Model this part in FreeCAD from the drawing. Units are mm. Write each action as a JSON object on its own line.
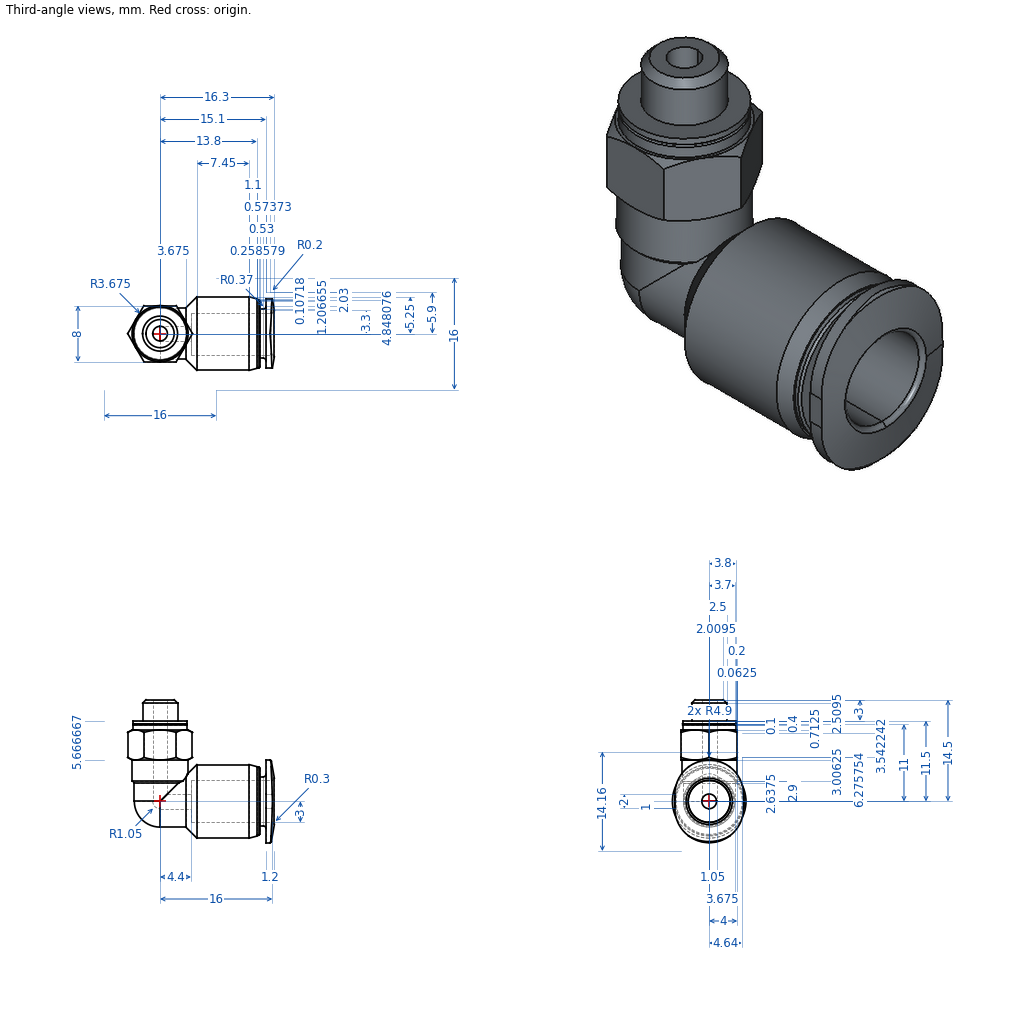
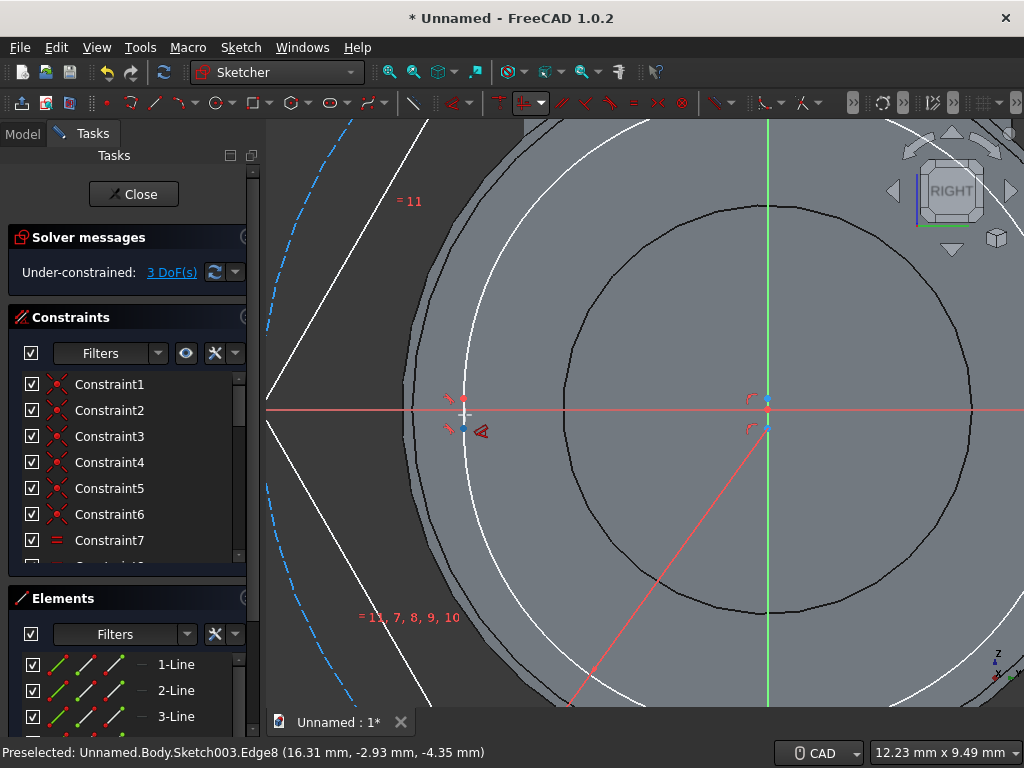
{"action": "left_click", "coordinate": [464, 414]}
{"action": "left_click", "coordinate": [430, 424]}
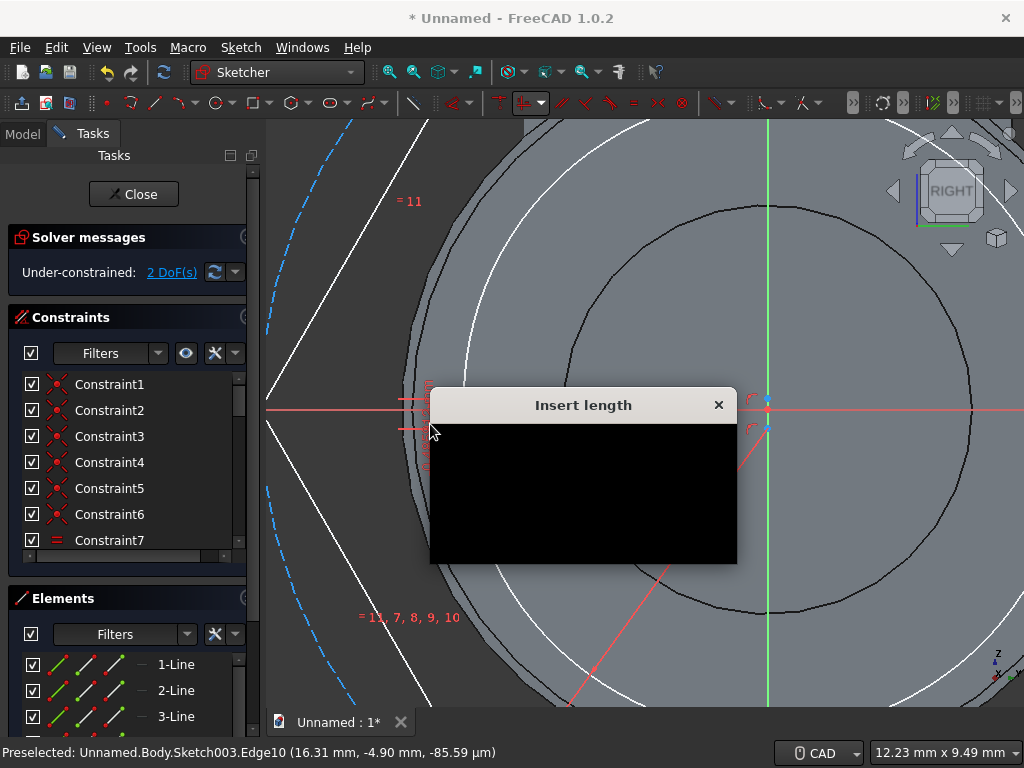
{"action": "type", "text": "2"}
{"action": "key", "text": "Return"}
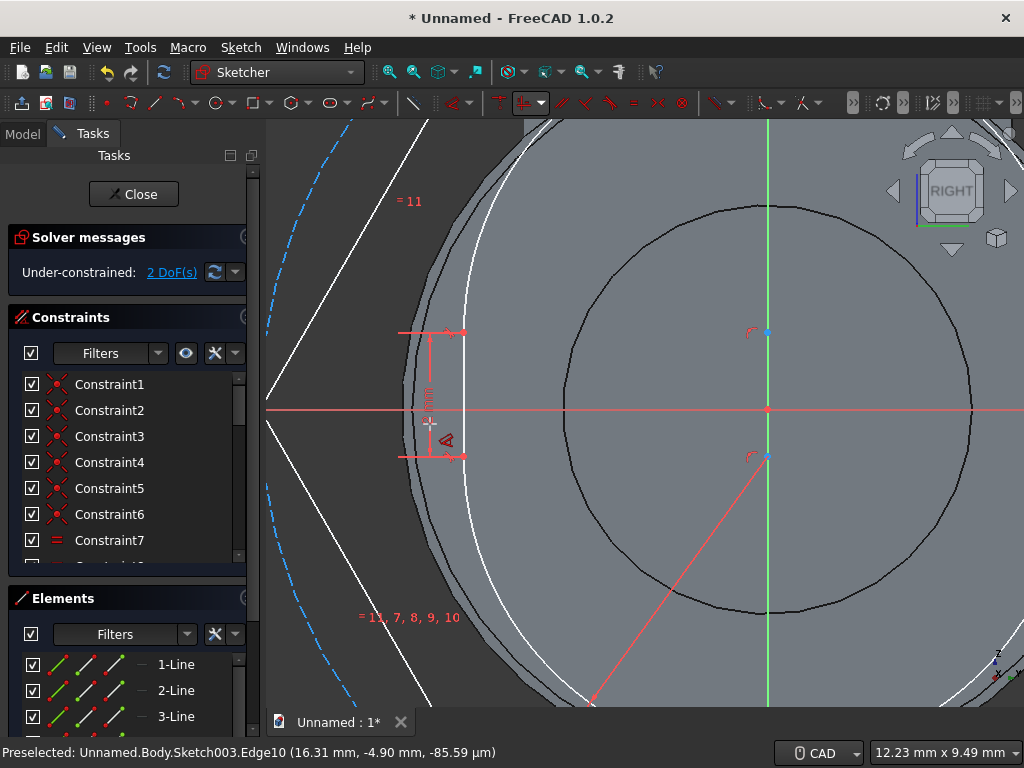
{"action": "left_click", "coordinate": [464, 457]}
{"action": "left_click", "coordinate": [430, 450]}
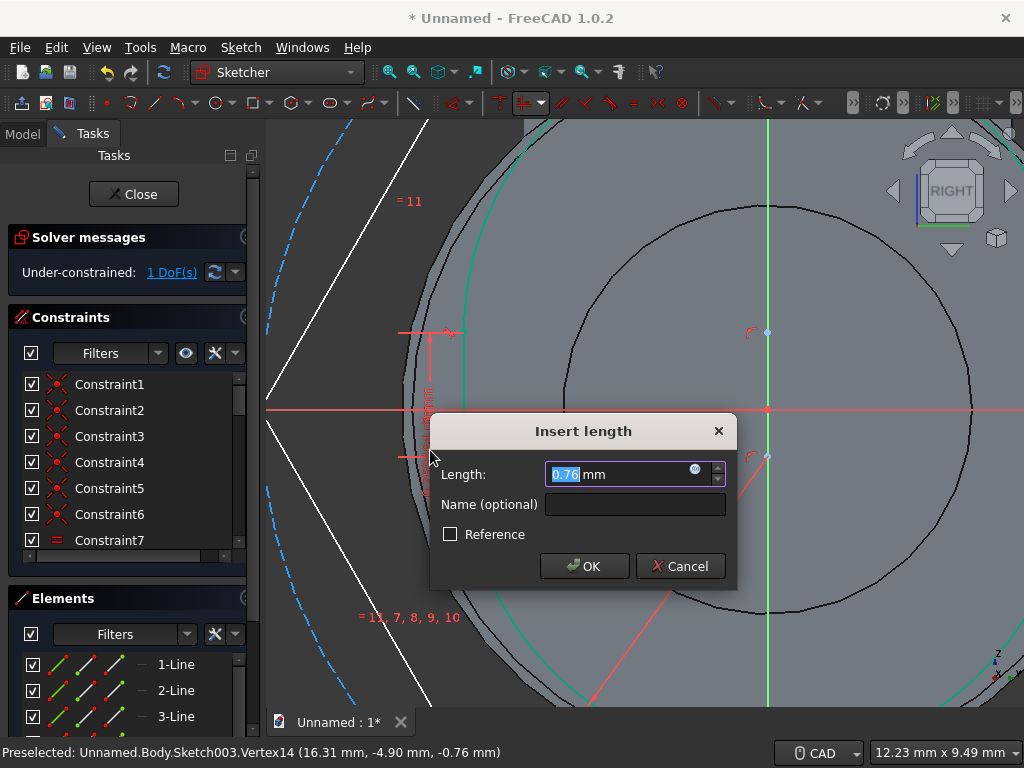
{"action": "type", "text": "1"}
{"action": "key", "text": "Return"}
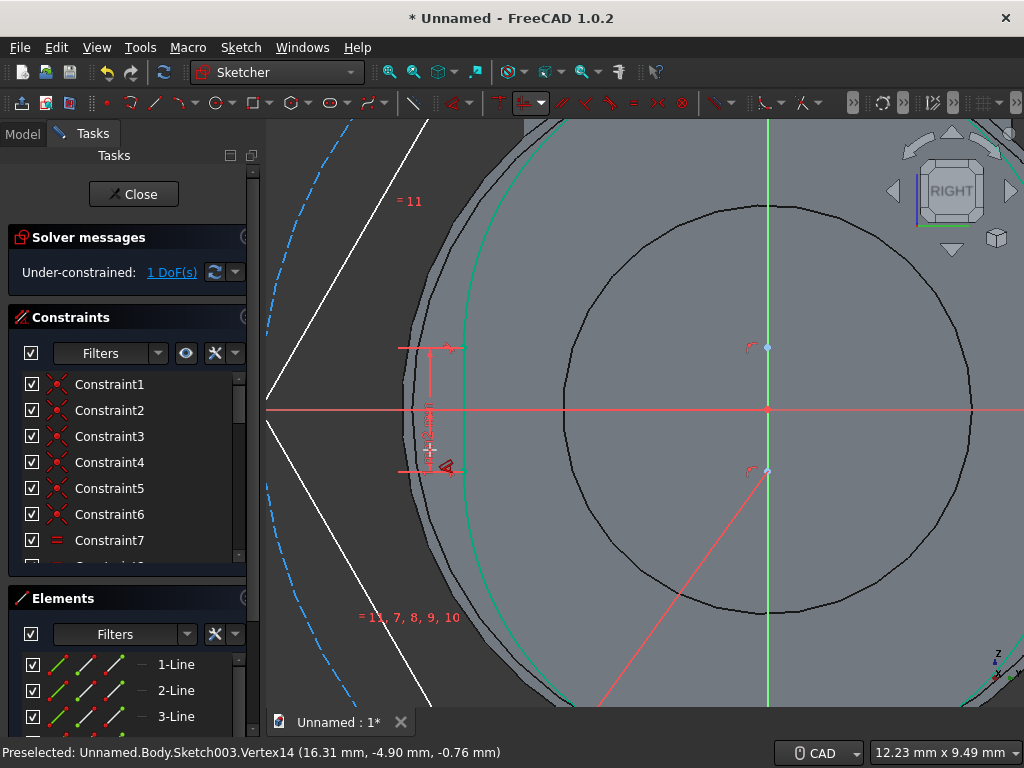
{"action": "scroll", "coordinate": [465, 415], "scroll_direction": "down", "scroll_amount": 5}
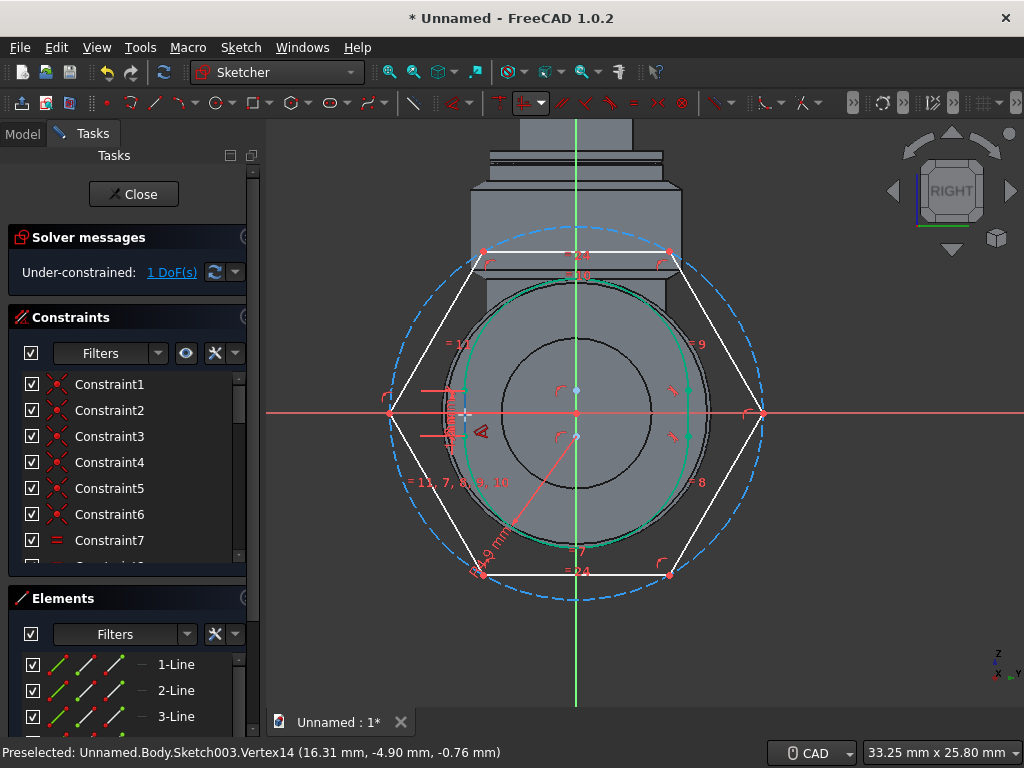
{"action": "left_click", "coordinate": [483, 575]}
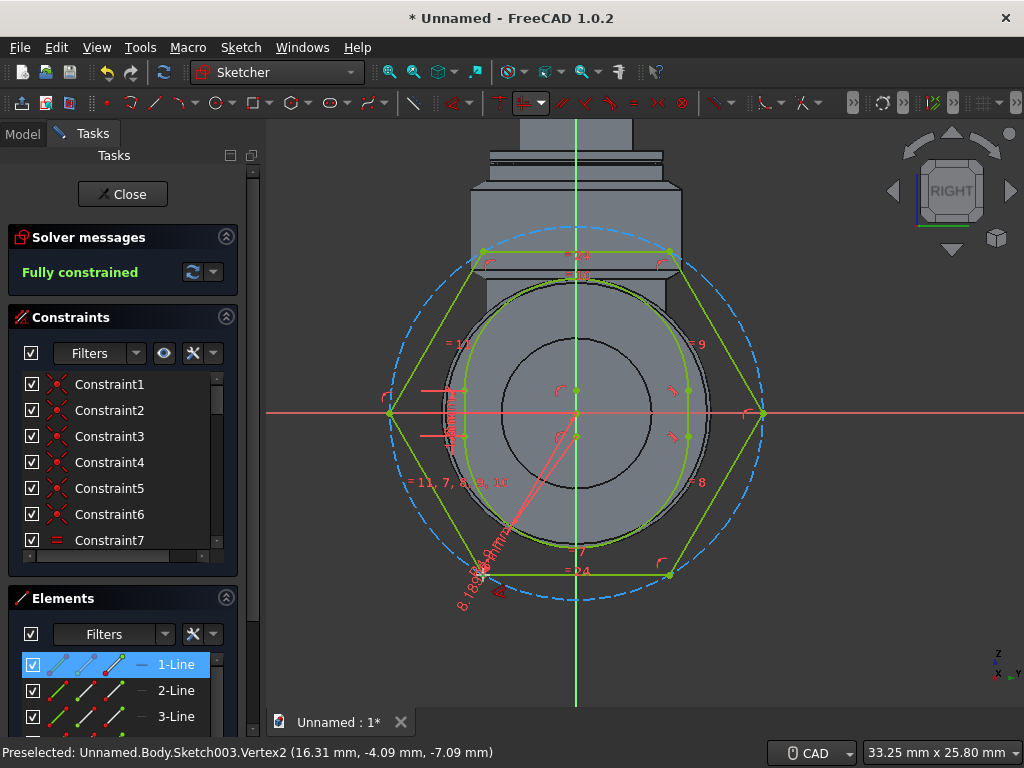
{"action": "left_click", "coordinate": [670, 252]}
{"action": "left_click", "coordinate": [704, 339]}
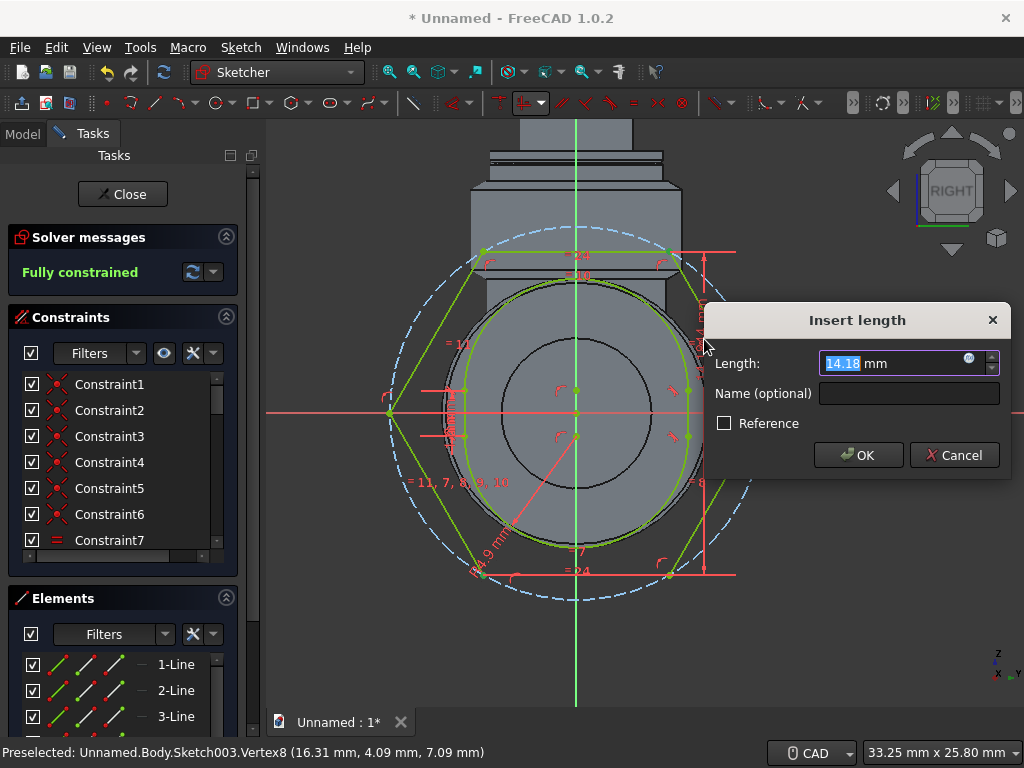
{"action": "type", "text": "14.16"}
{"action": "key", "text": "Return"}
{"action": "key", "text": "Escape"}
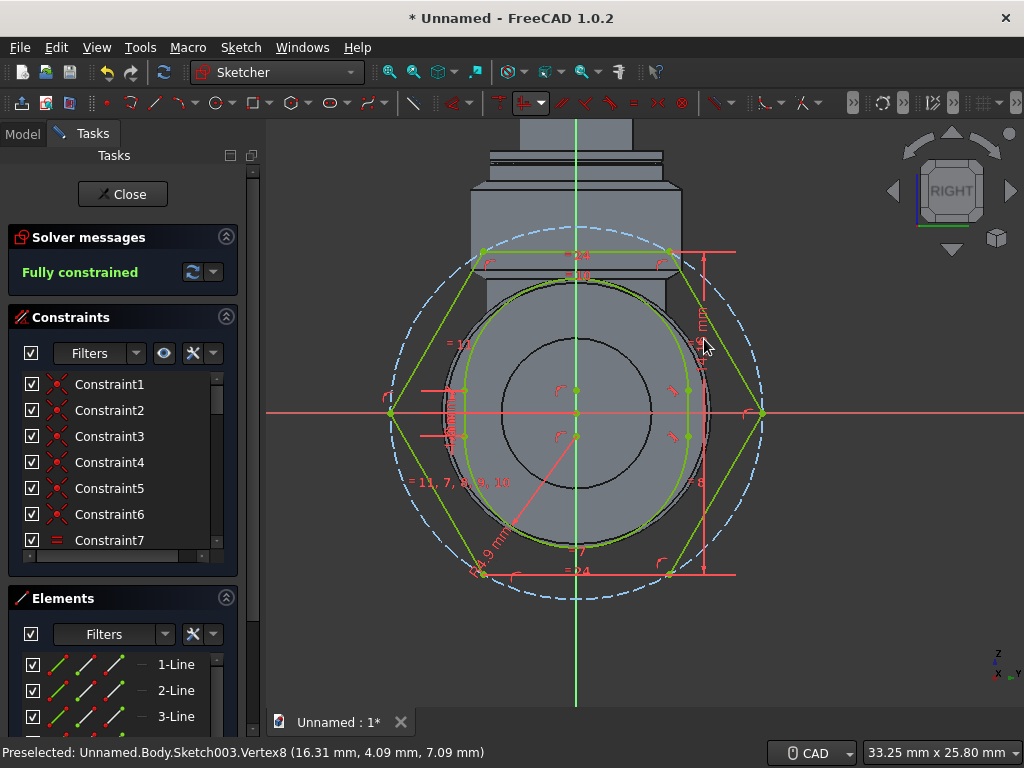
{"action": "left_click", "coordinate": [123, 194]}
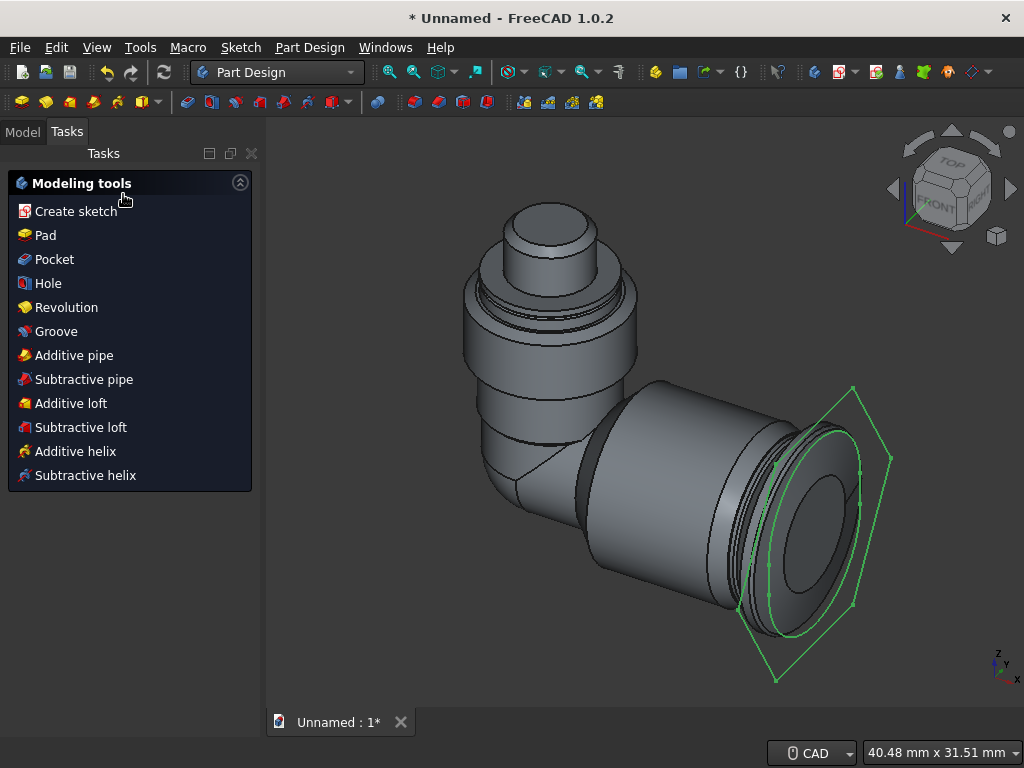
{"action": "left_click", "coordinate": [188, 102]}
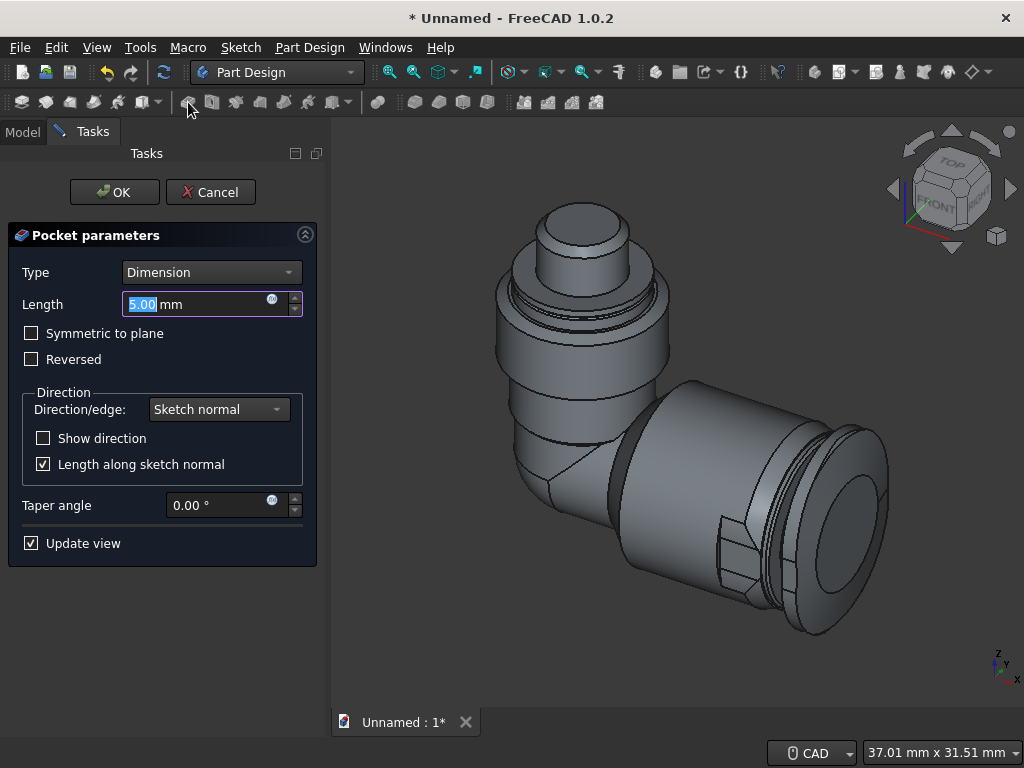
{"action": "type", "text": "1.2"}
{"action": "key", "text": "Tab"}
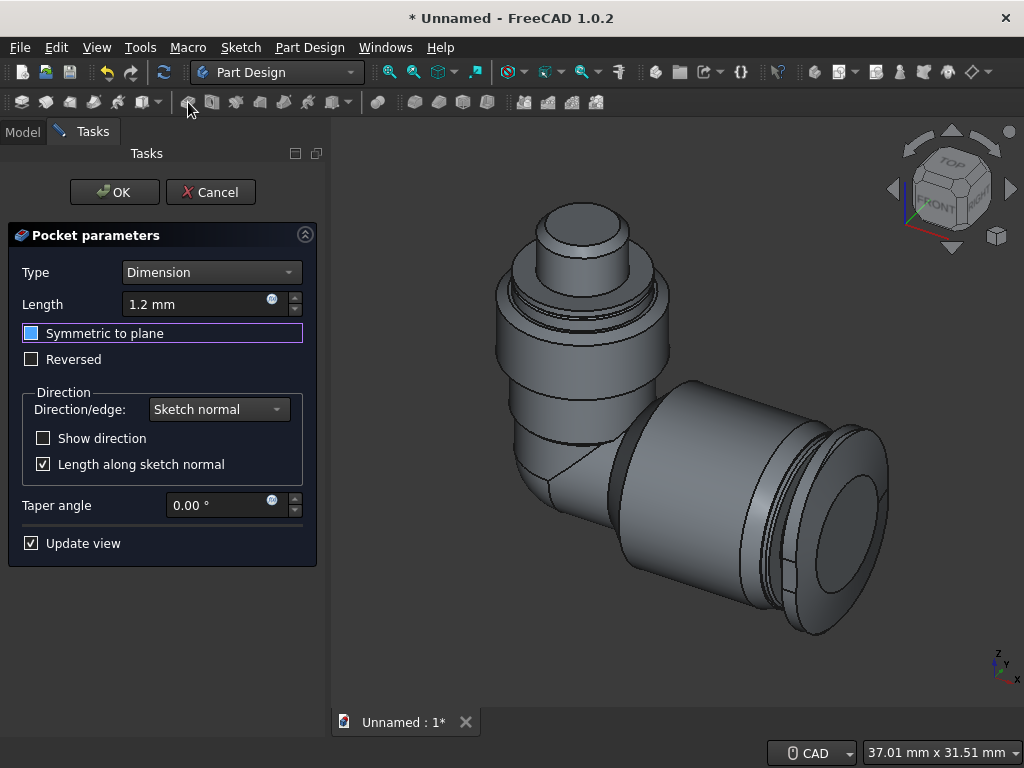
{"action": "left_click", "coordinate": [115, 192]}